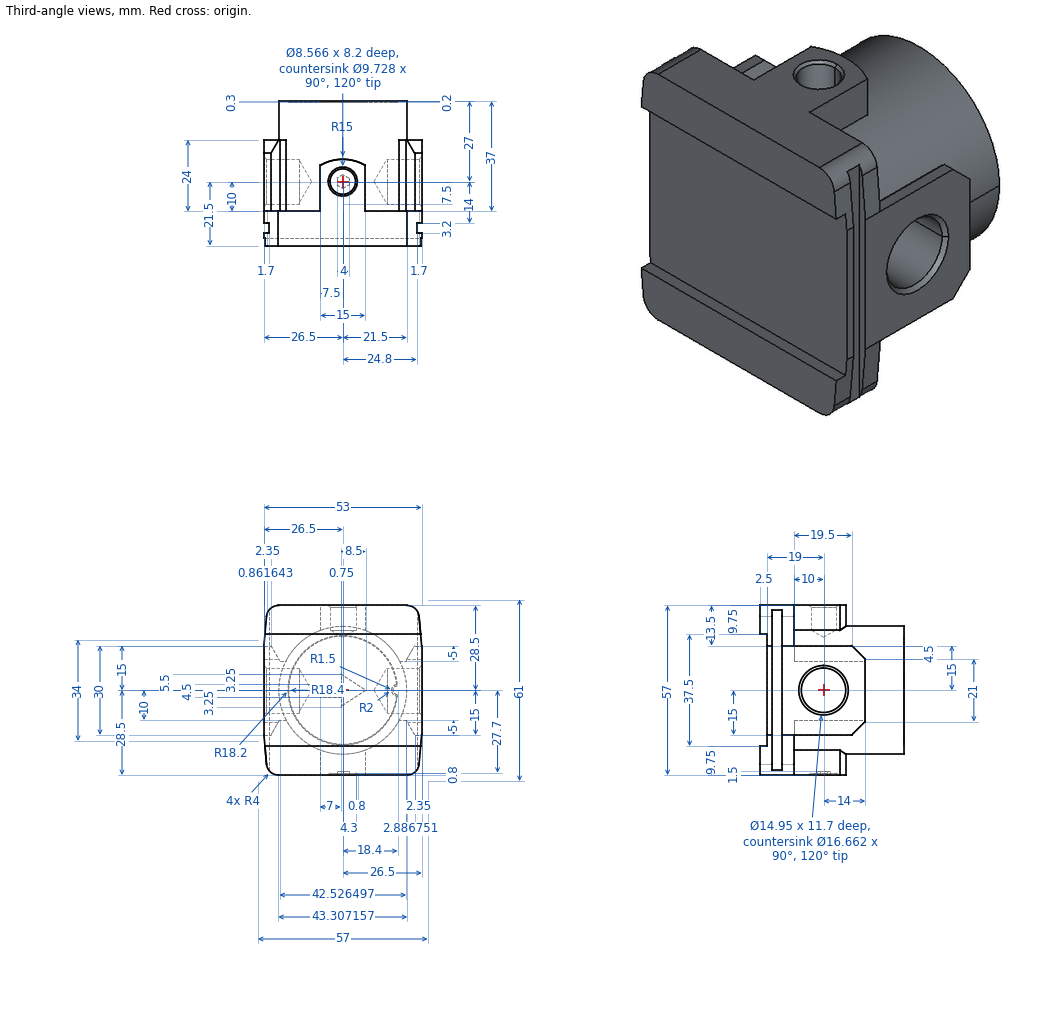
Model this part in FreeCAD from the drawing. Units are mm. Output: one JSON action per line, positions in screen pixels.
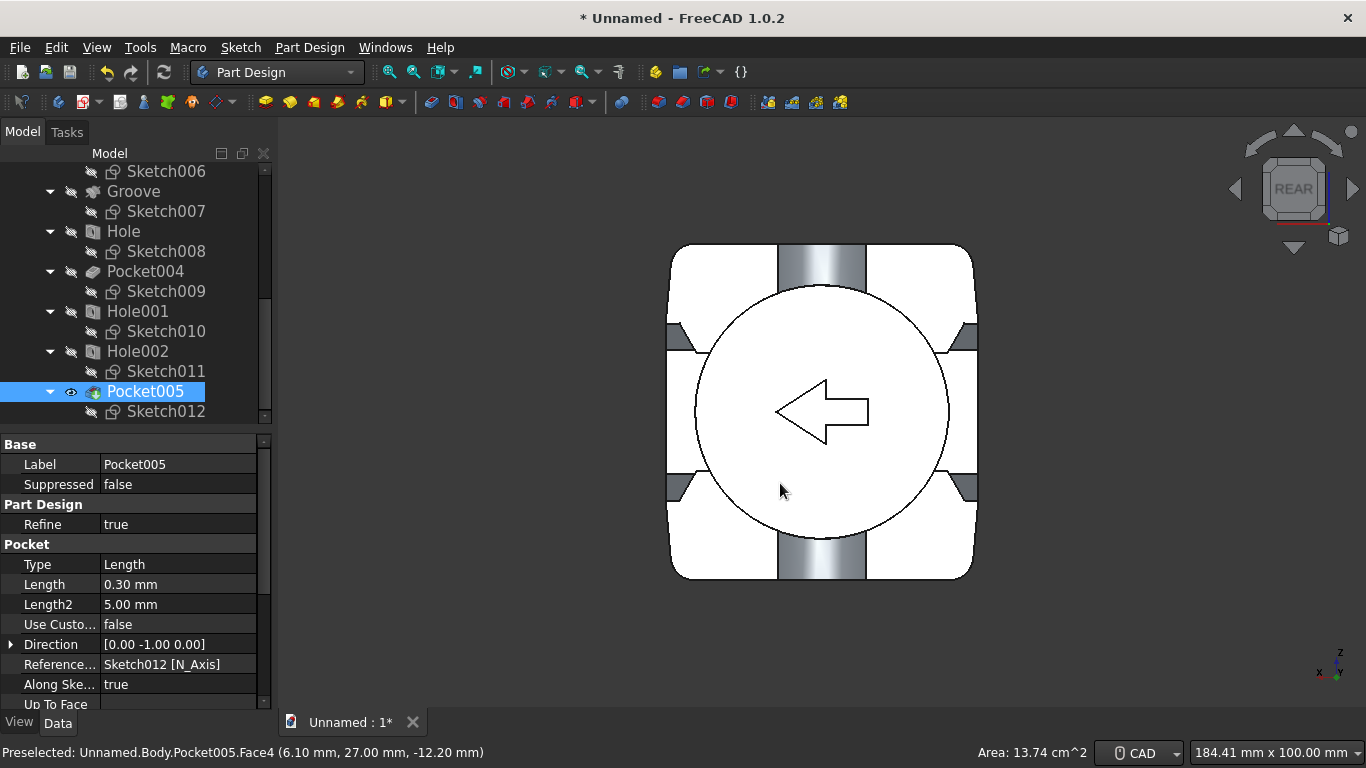
{"action": "left_click", "coordinate": [84, 102]}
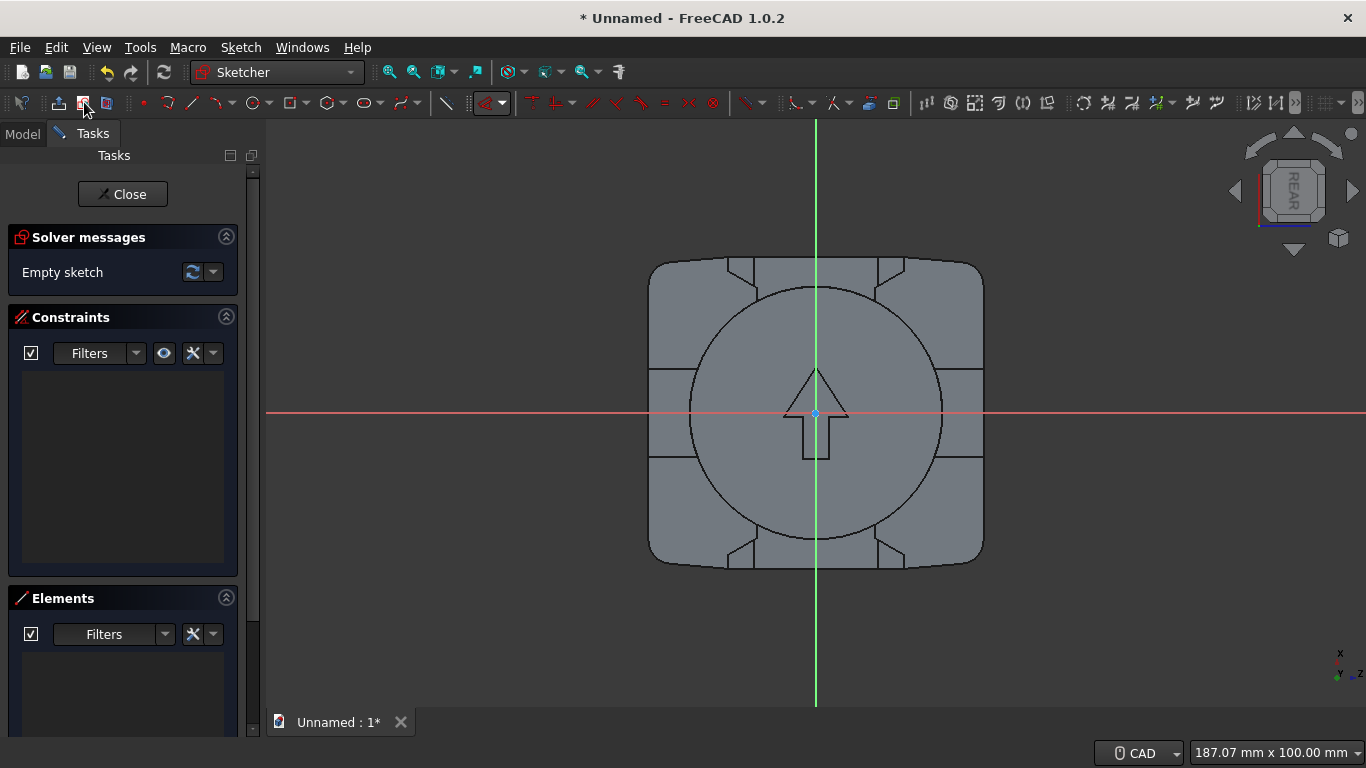
{"action": "scroll", "coordinate": [899, 413], "scroll_direction": "up", "scroll_amount": 3}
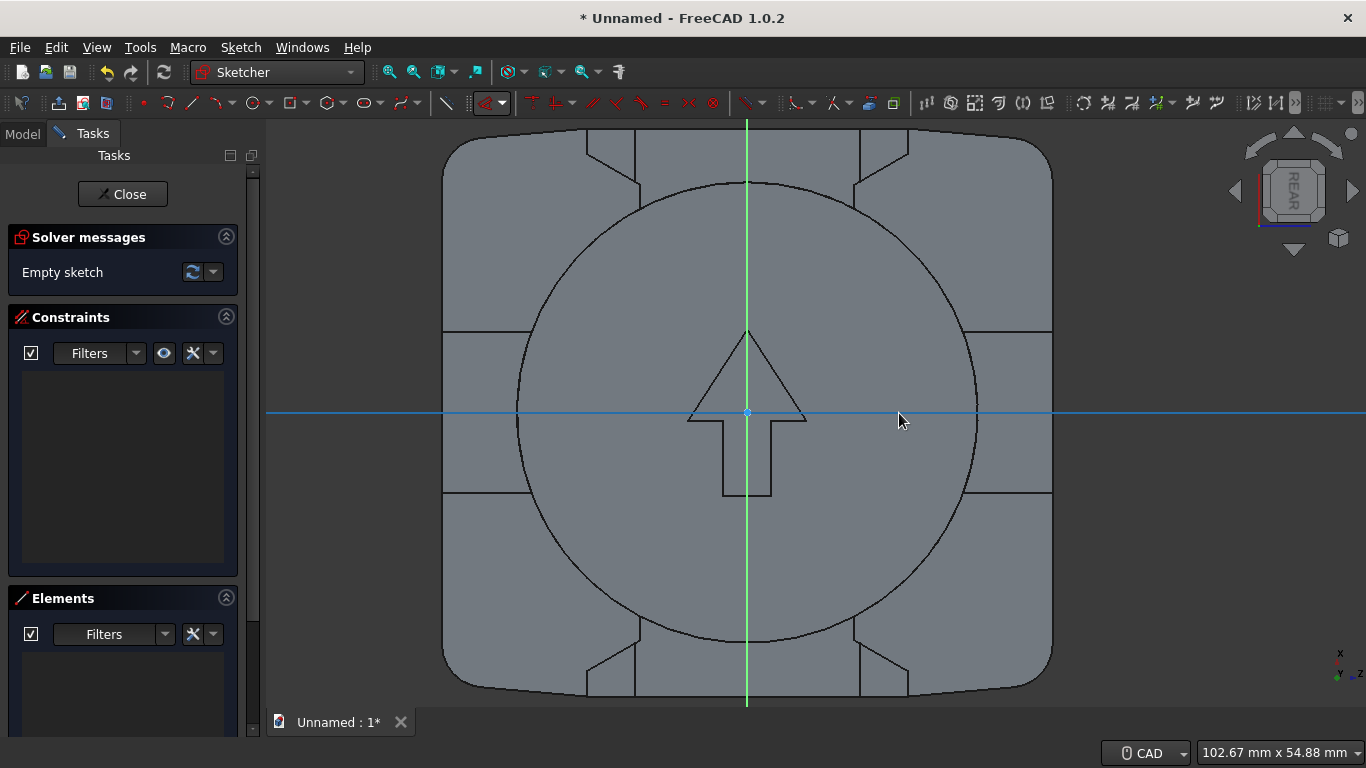
{"action": "key", "text": "g 3 a"}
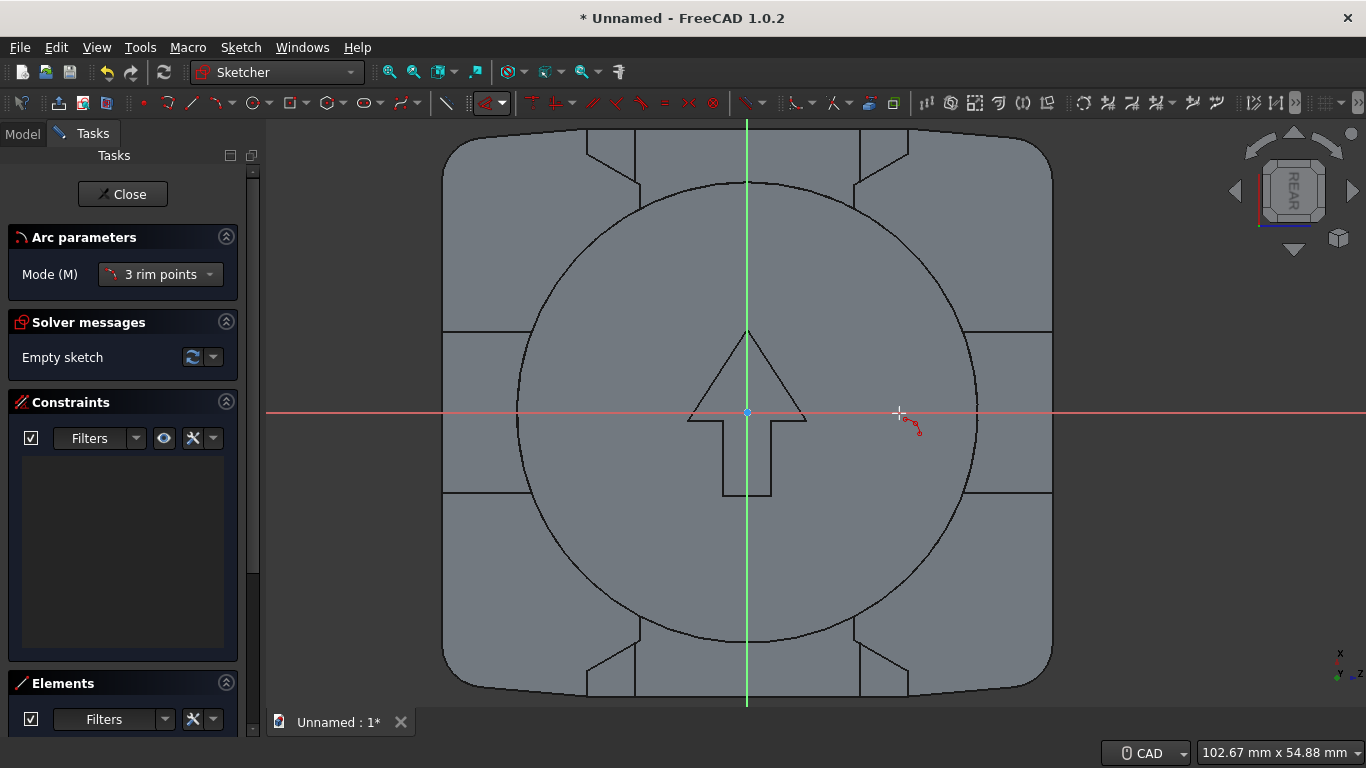
{"action": "left_click", "coordinate": [731, 216]}
{"action": "left_click", "coordinate": [763, 216]}
{"action": "left_click", "coordinate": [634, 574]}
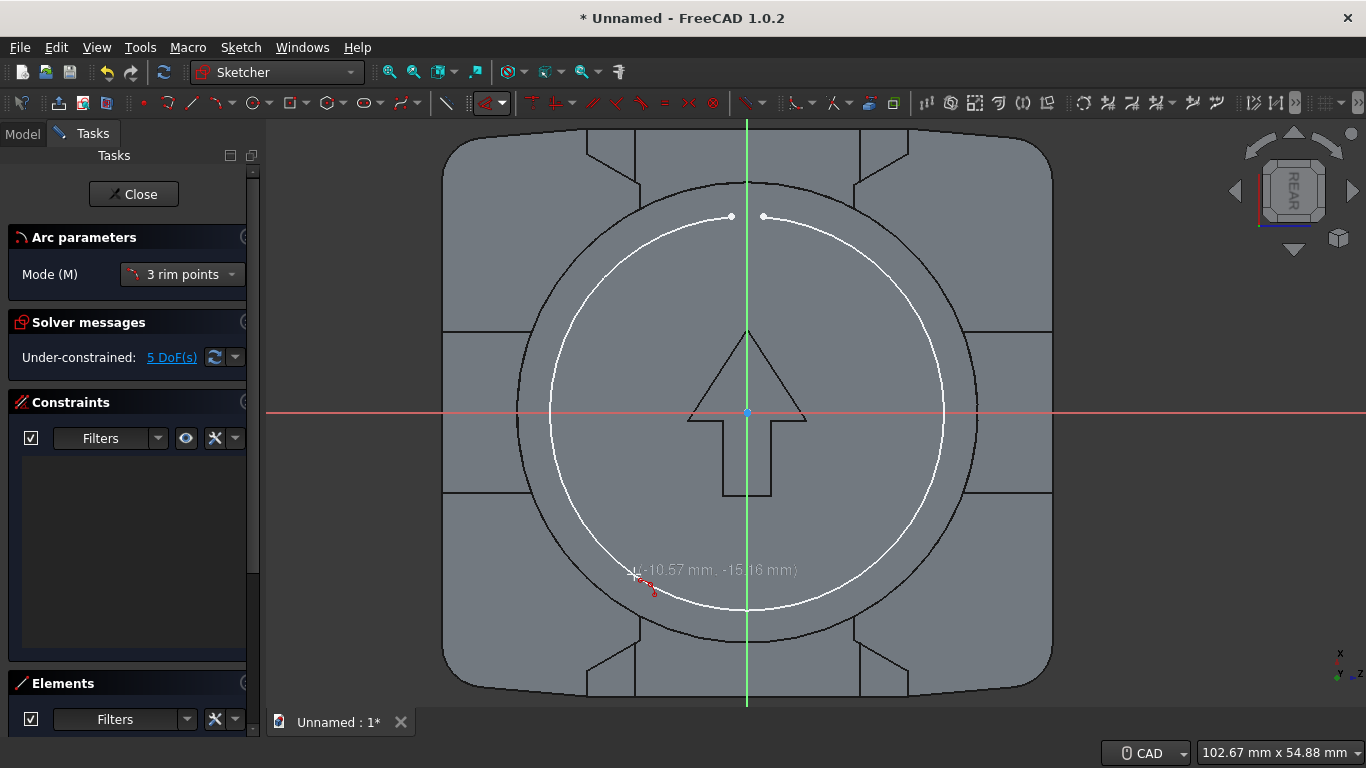
{"action": "left_click", "coordinate": [763, 217]}
{"action": "left_click", "coordinate": [731, 217]}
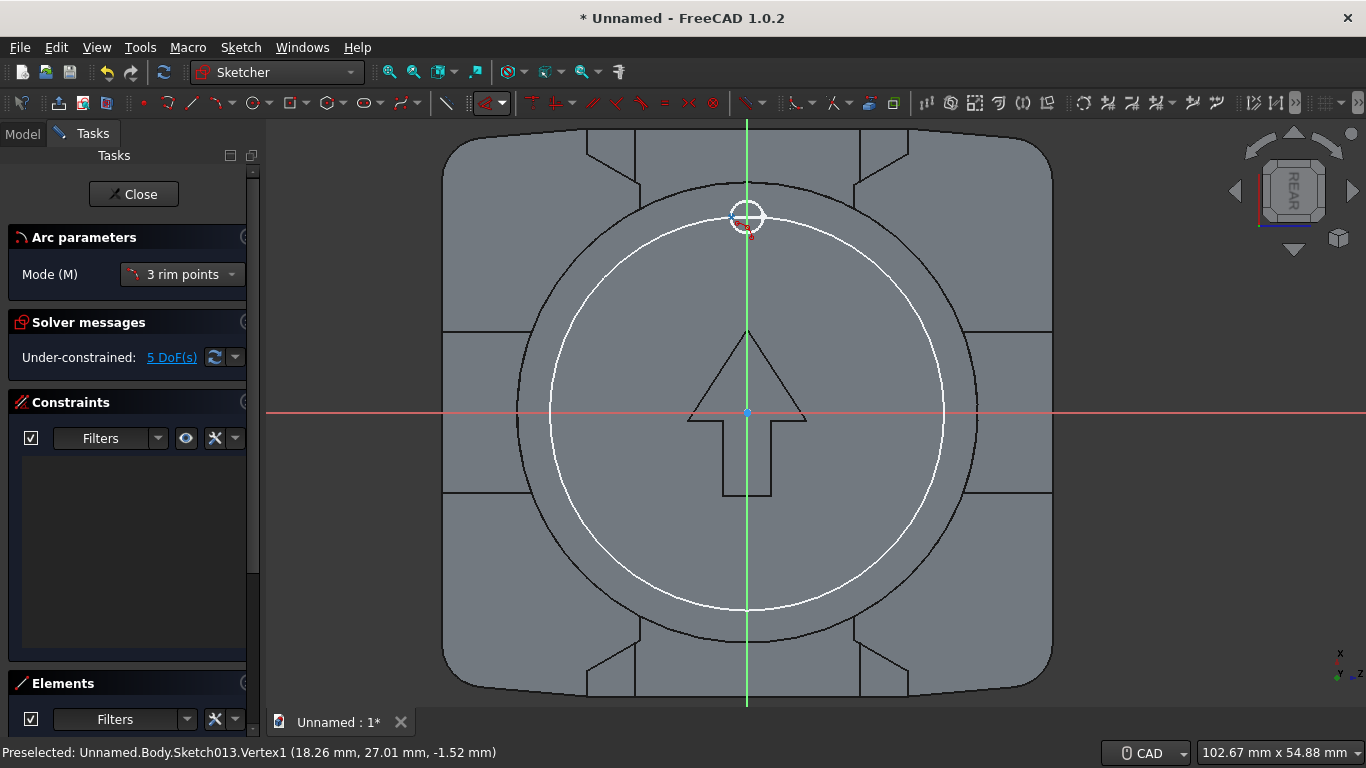
{"action": "scroll", "coordinate": [738, 229], "scroll_direction": "up", "scroll_amount": 3}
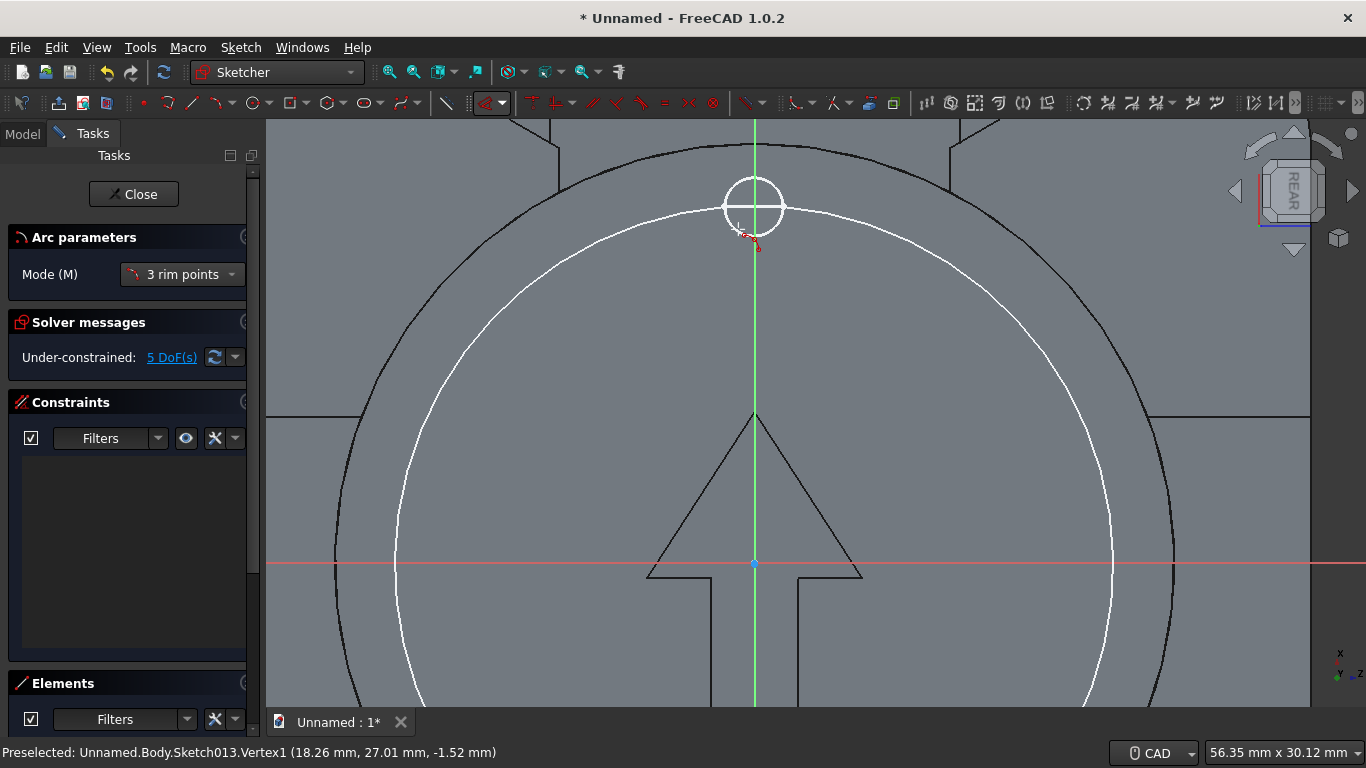
{"action": "left_click", "coordinate": [738, 228]}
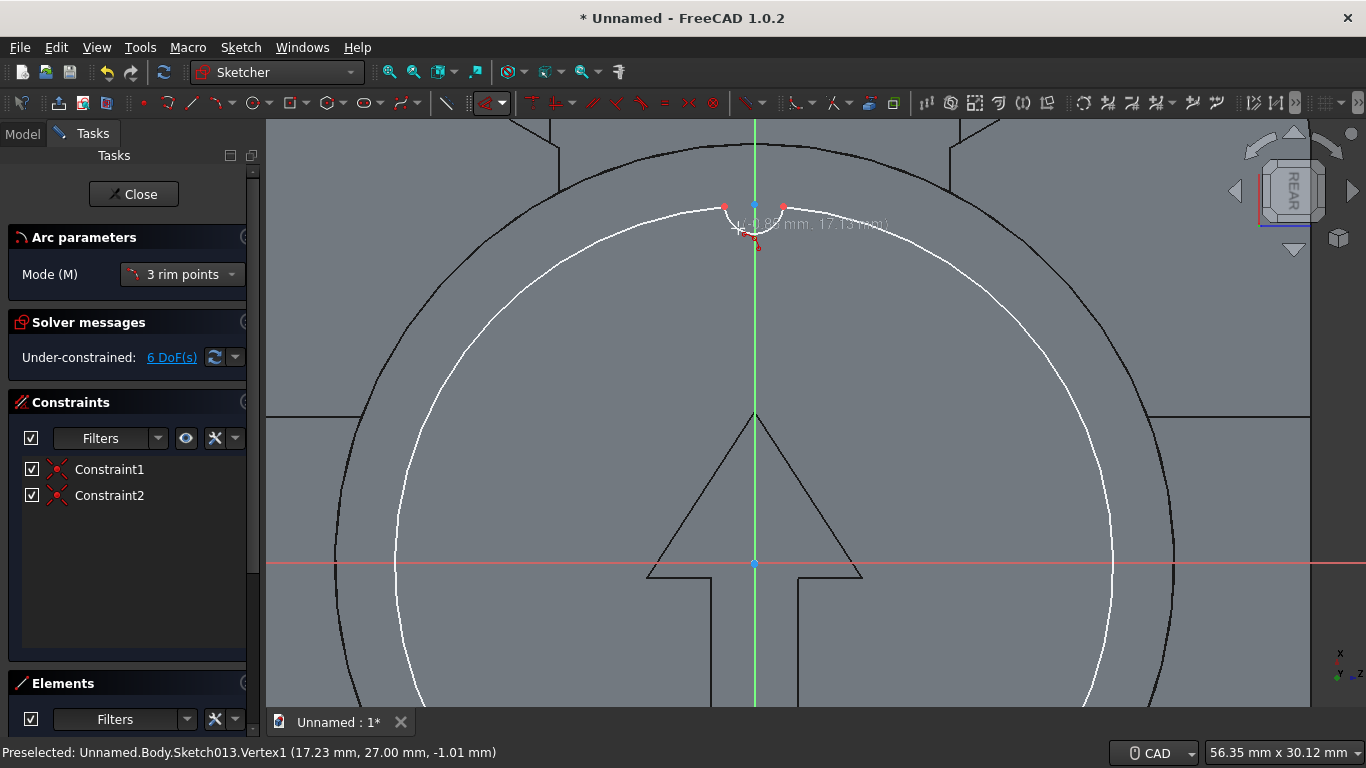
{"action": "scroll", "coordinate": [716, 210], "scroll_direction": "up", "scroll_amount": 8}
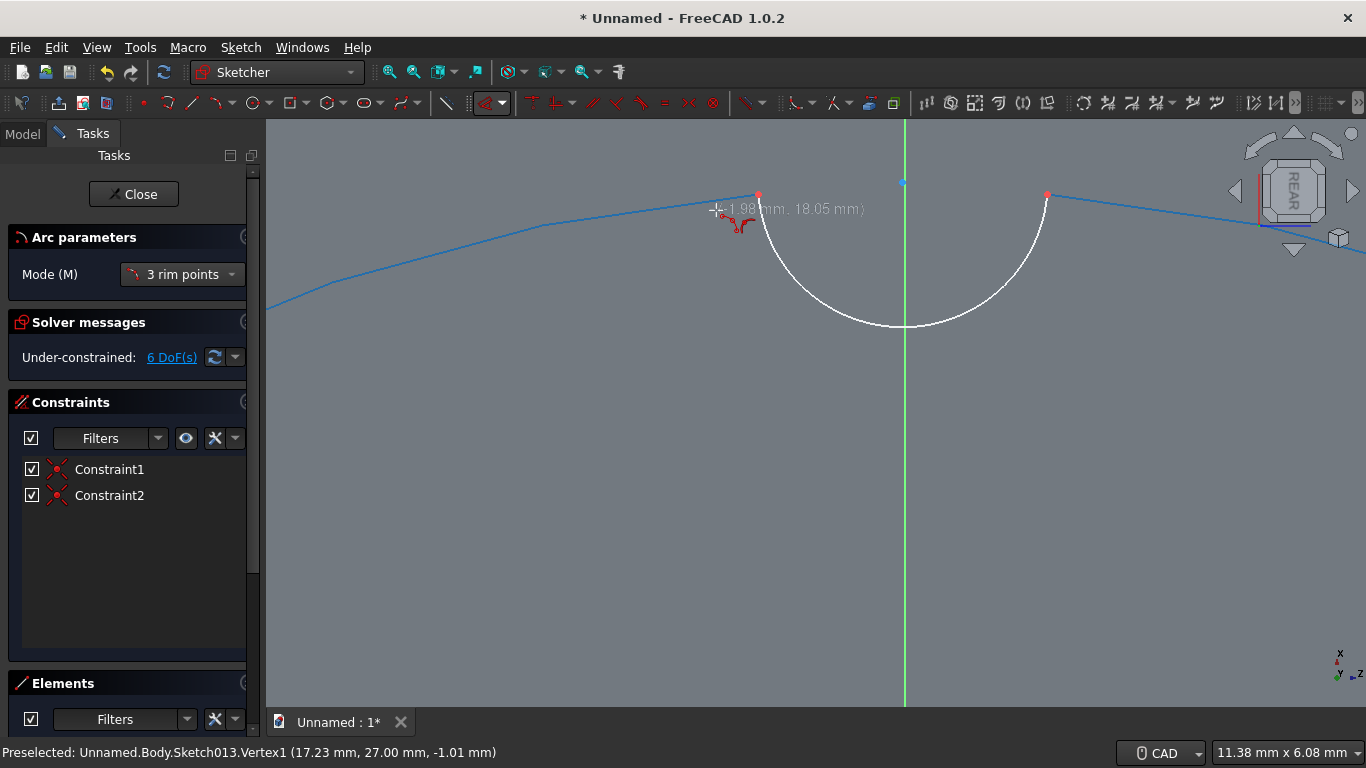
{"action": "left_click", "coordinate": [714, 210]}
{"action": "left_click", "coordinate": [1097, 210]}